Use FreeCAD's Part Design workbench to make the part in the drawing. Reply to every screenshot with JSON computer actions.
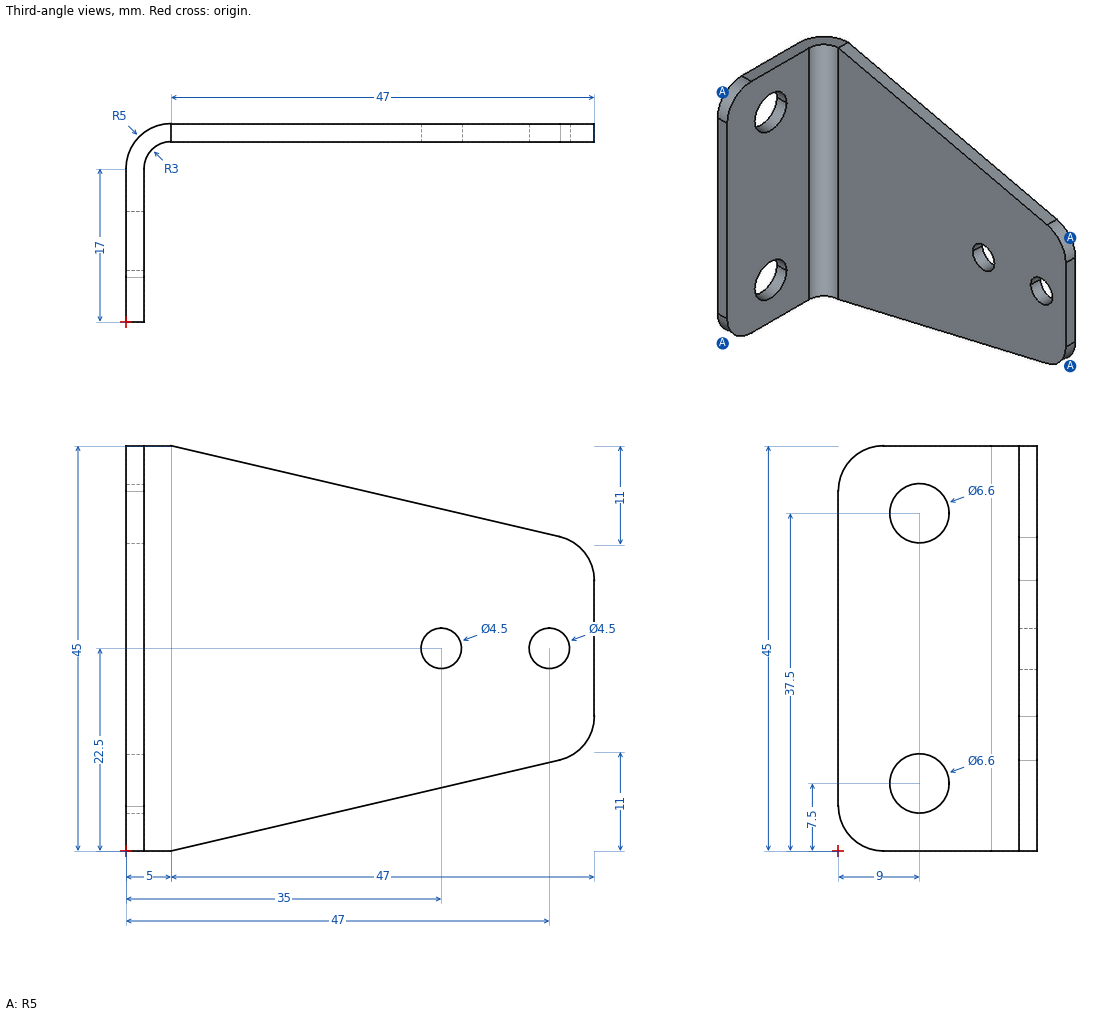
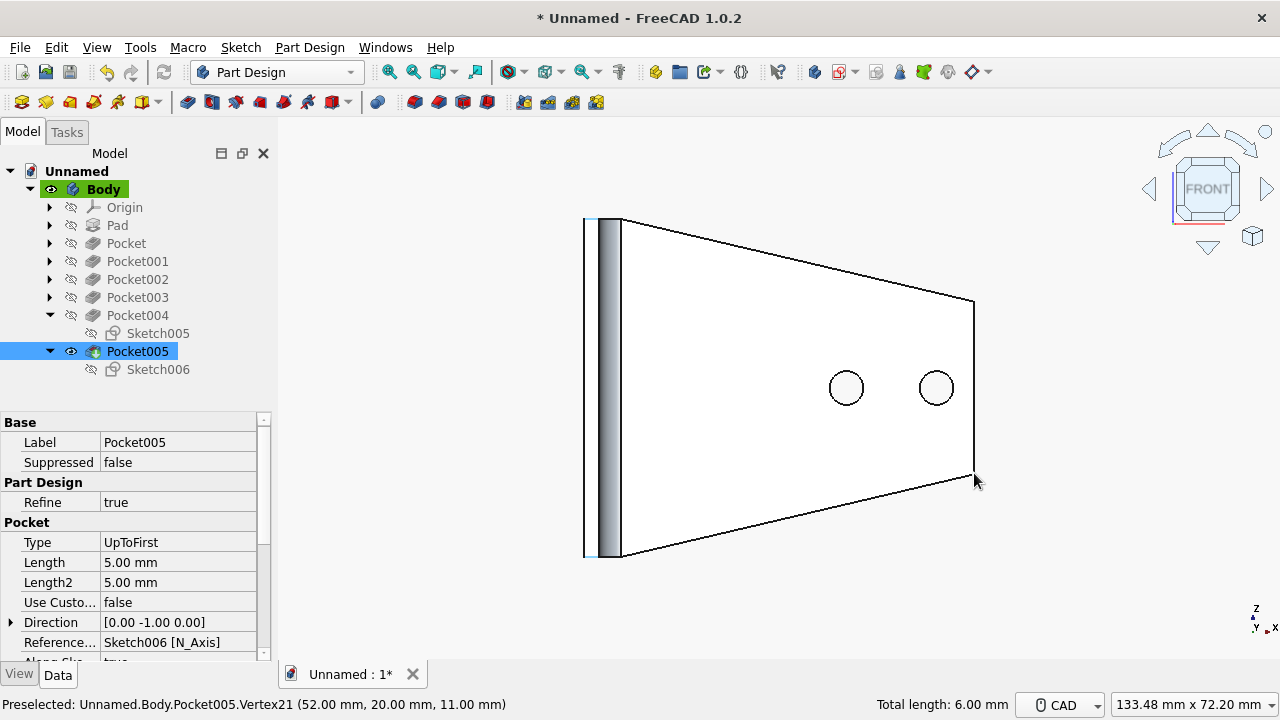
{"action": "key", "text": "3"}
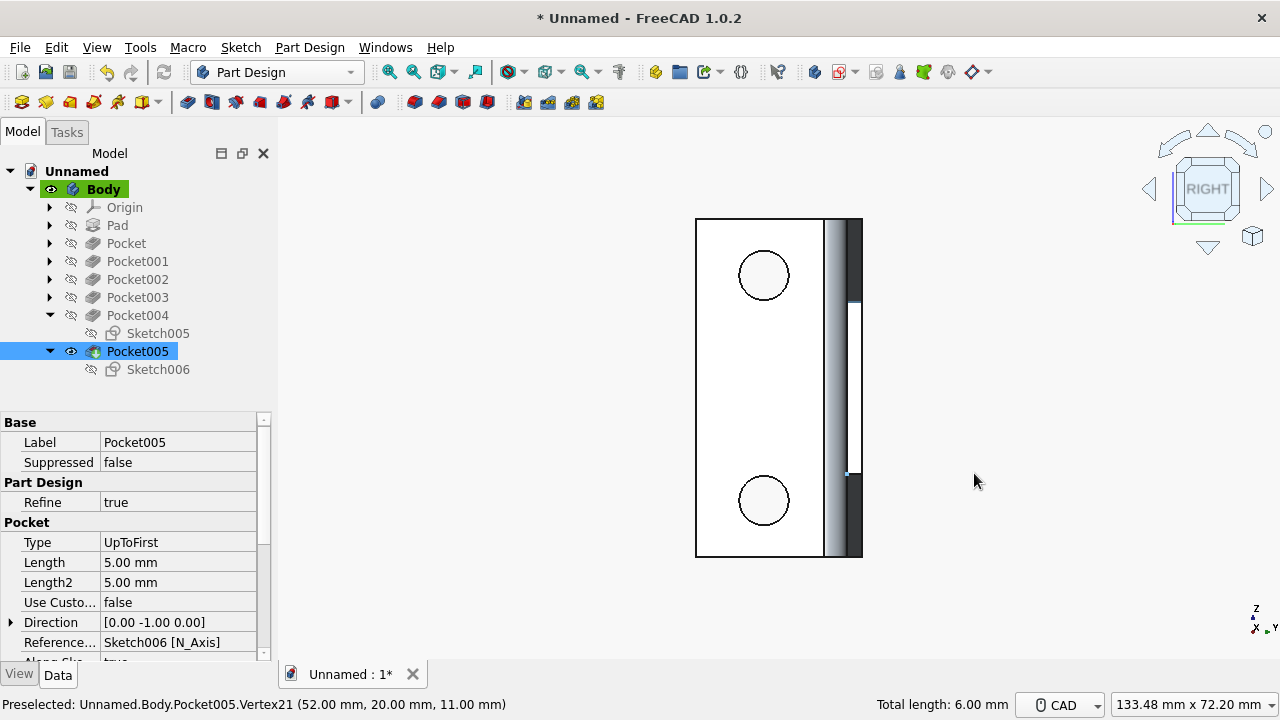
{"action": "left_click", "coordinate": [854, 473], "text": "ctrl"}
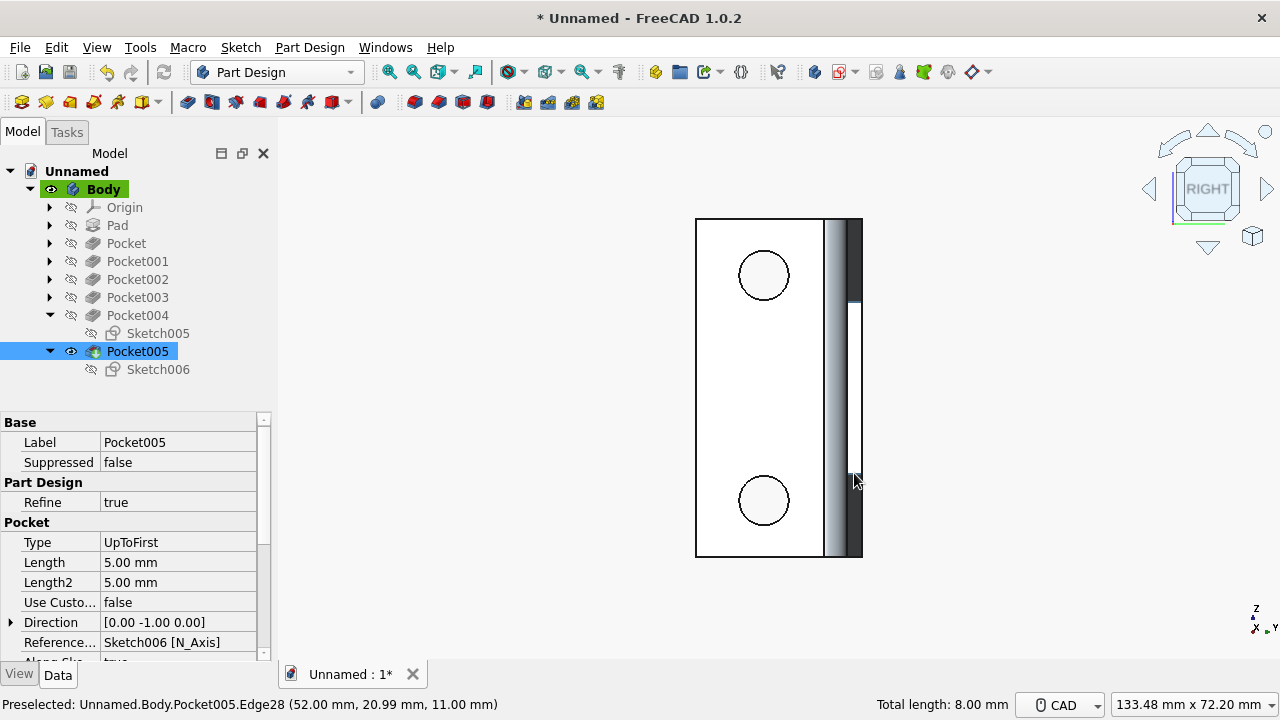
{"action": "left_click", "coordinate": [416, 102]}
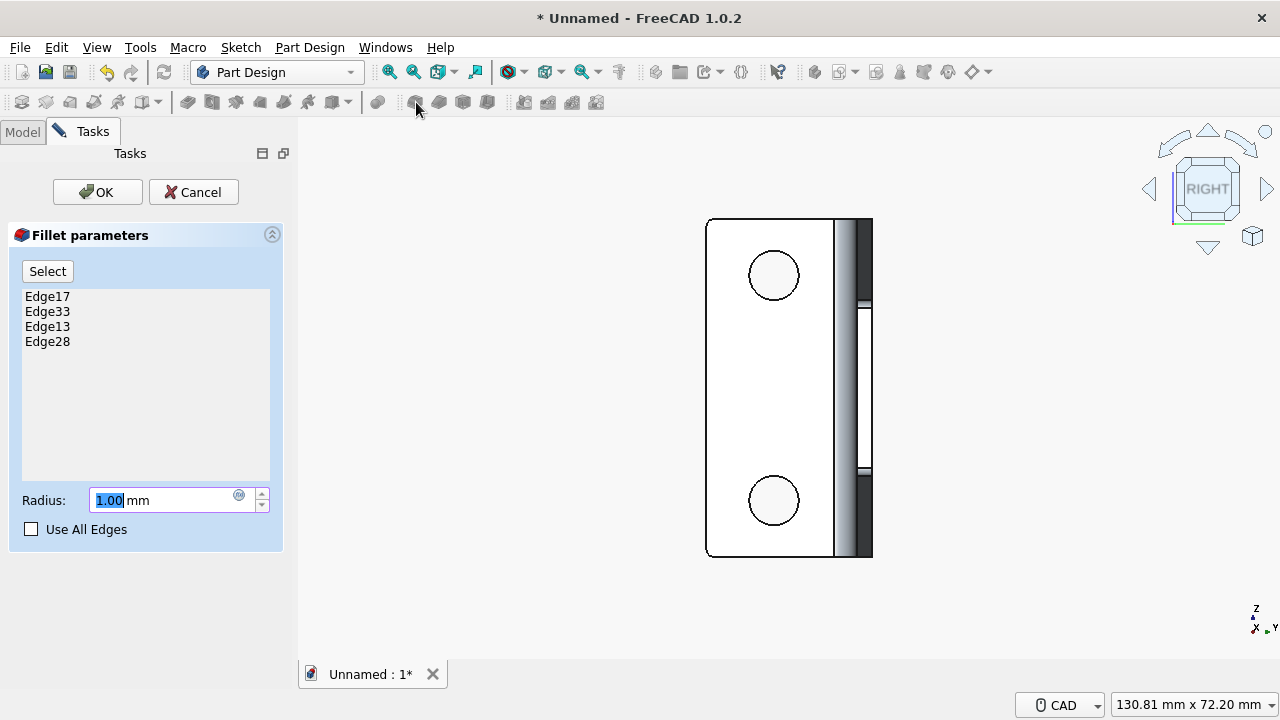
{"action": "type", "text": "5"}
{"action": "key", "text": "Tab"}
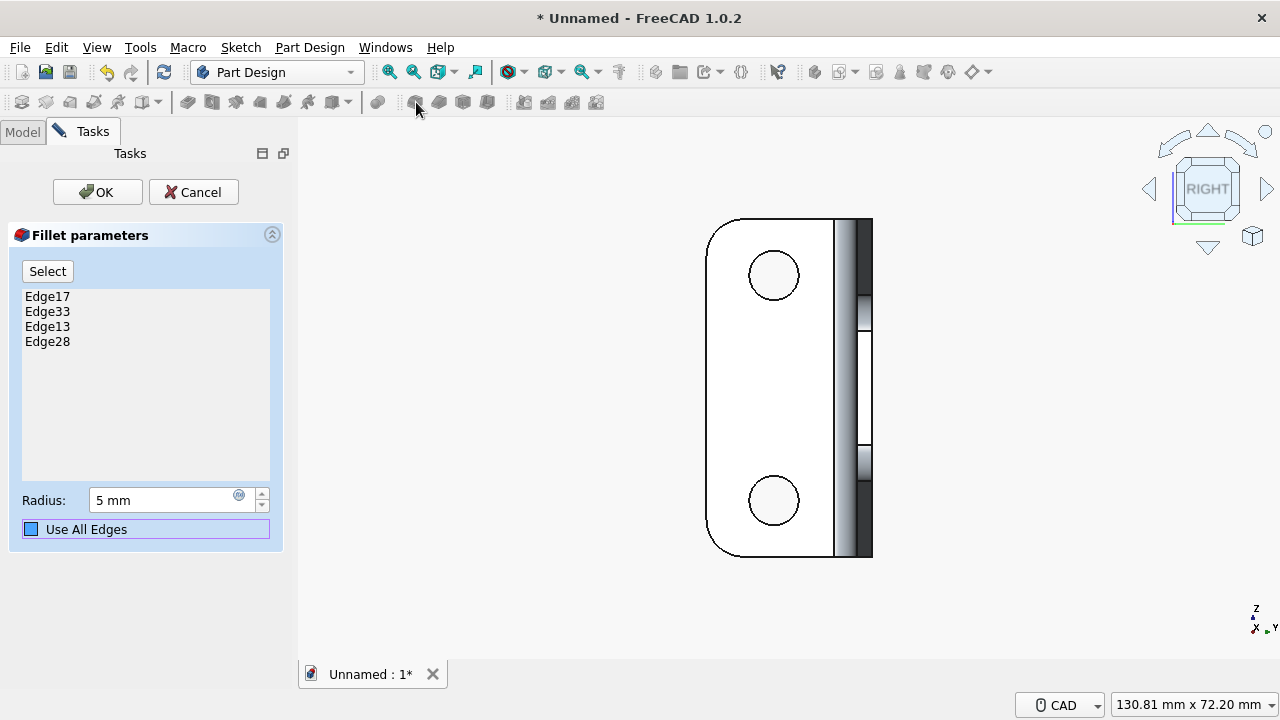
{"action": "left_click", "coordinate": [98, 192]}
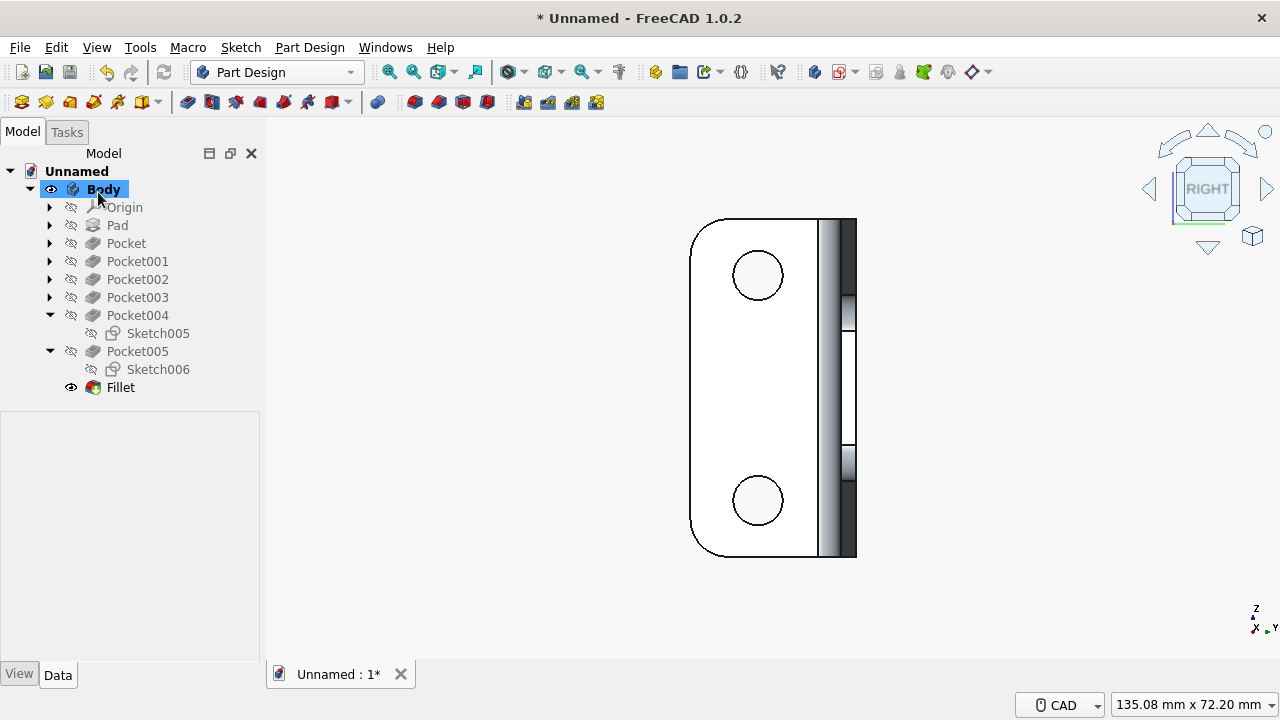
{"action": "key", "text": "0"}